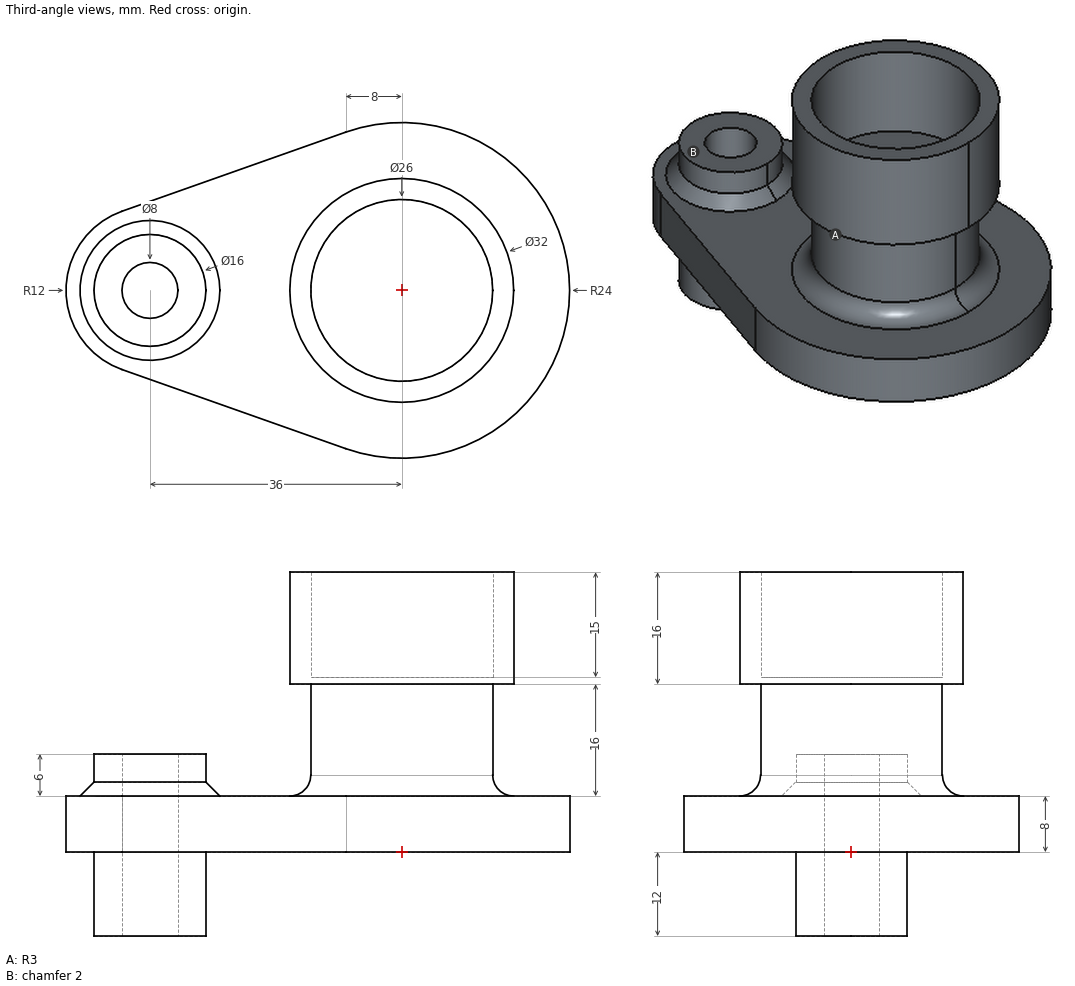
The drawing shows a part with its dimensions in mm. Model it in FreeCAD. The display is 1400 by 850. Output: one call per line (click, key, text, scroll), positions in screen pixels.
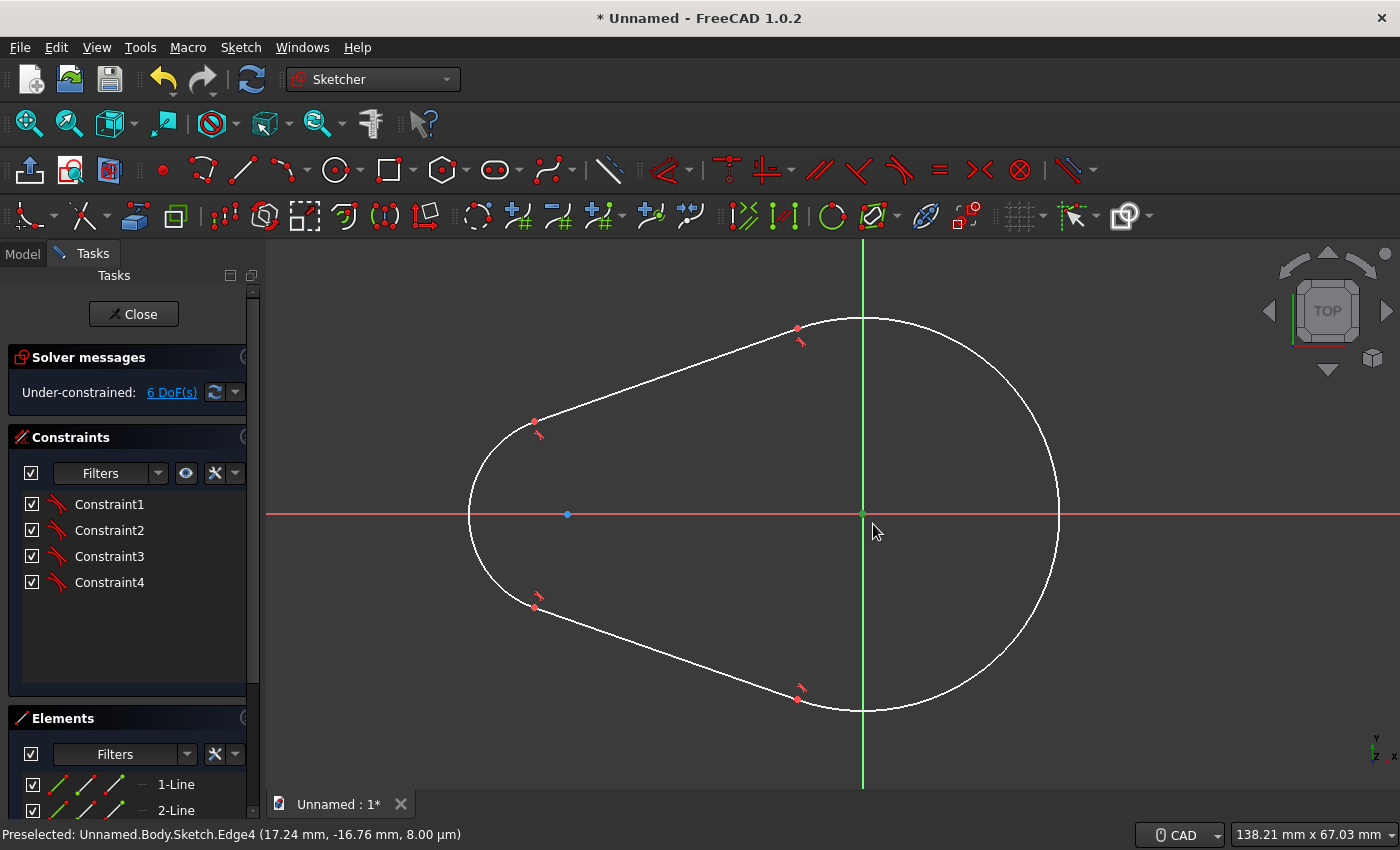
key(c)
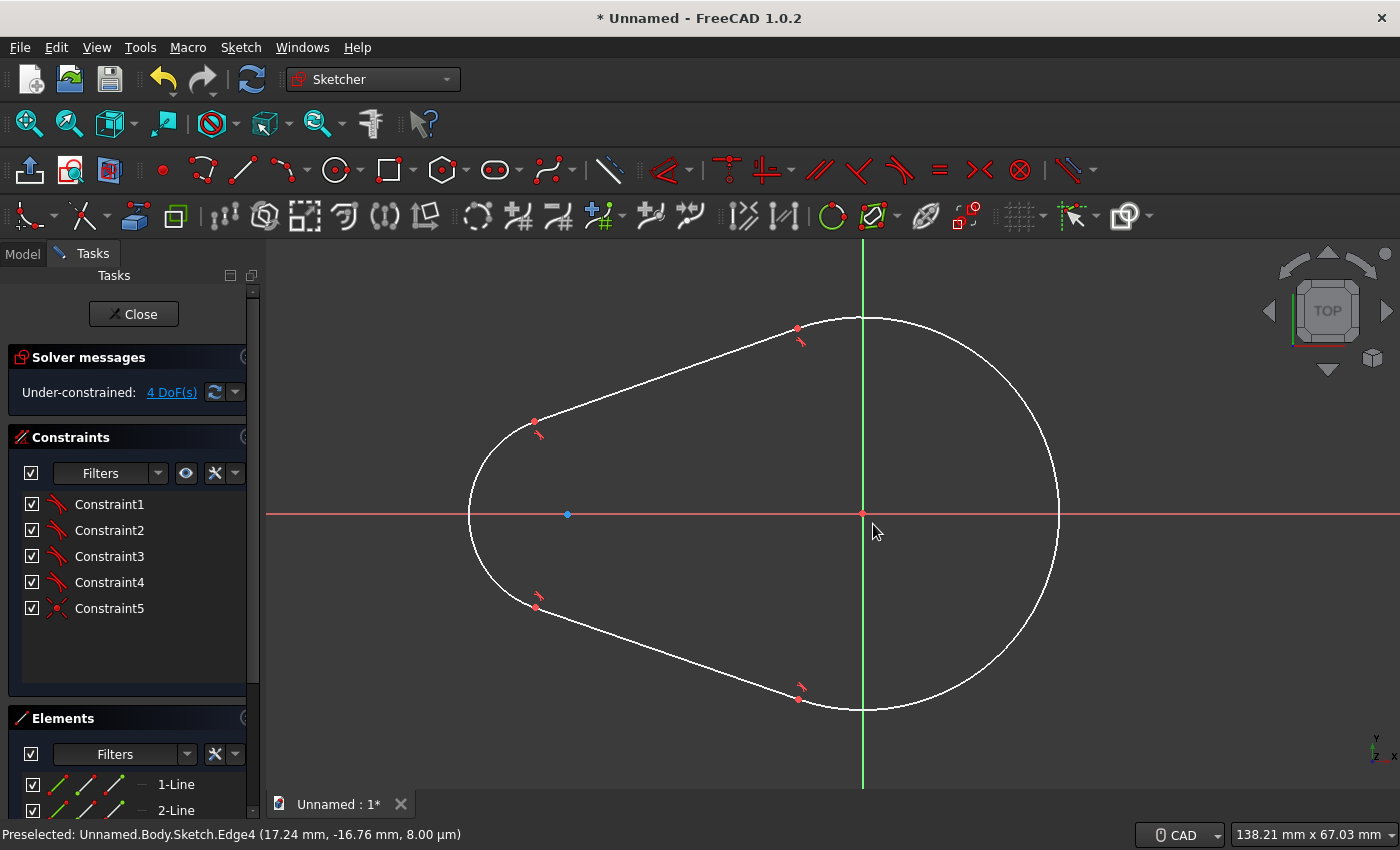
click(568, 515)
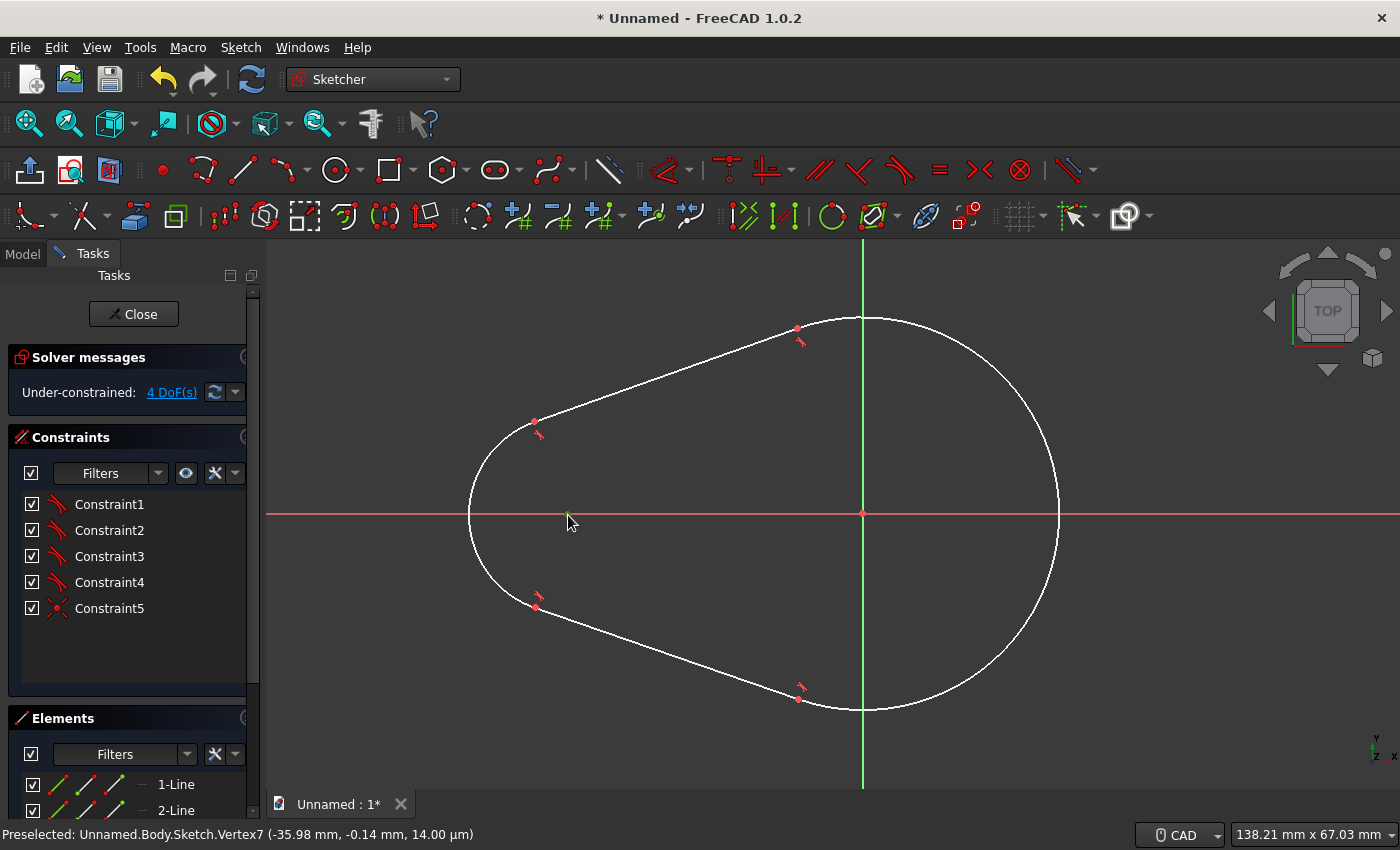
click(361, 514)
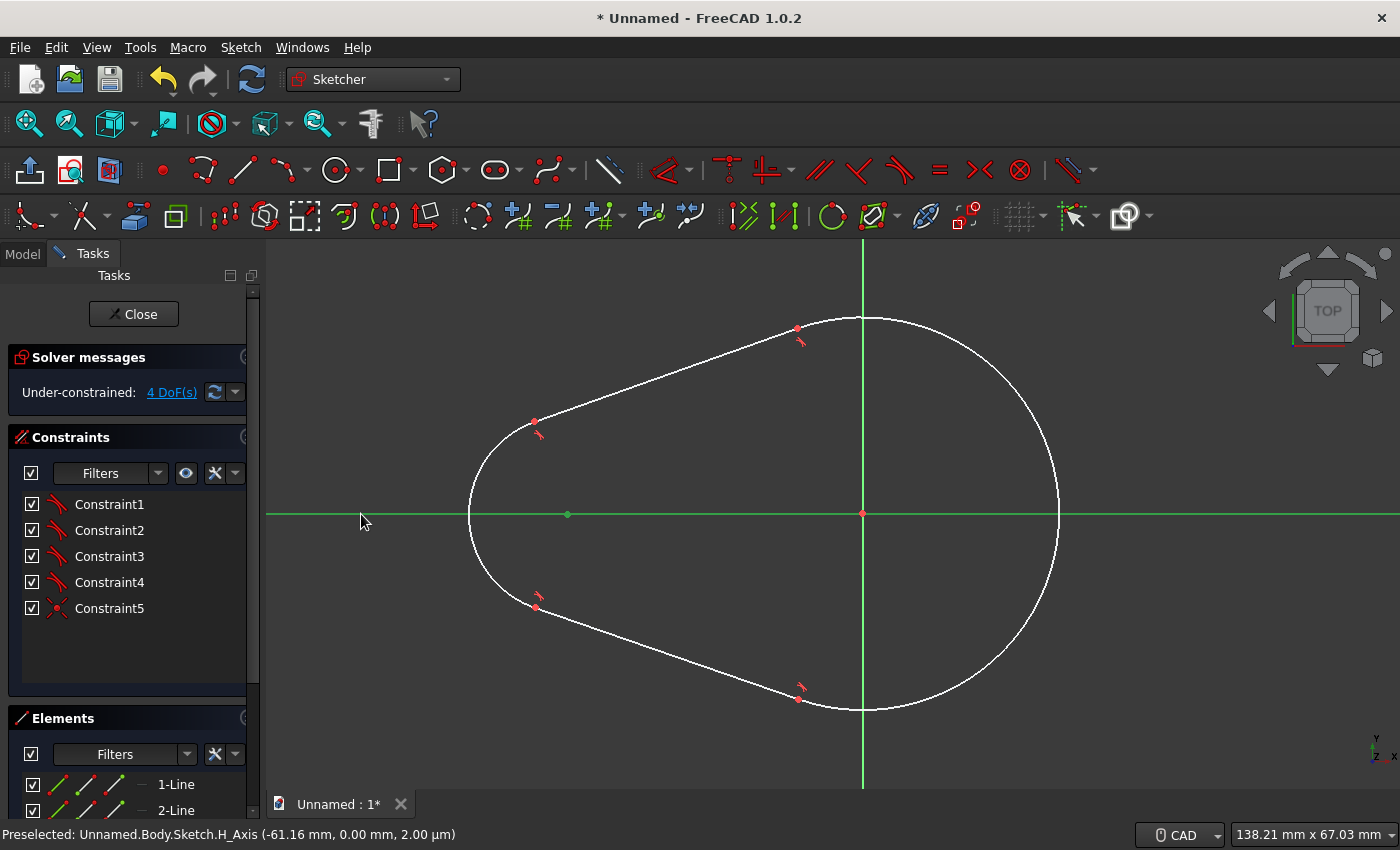
click(728, 170)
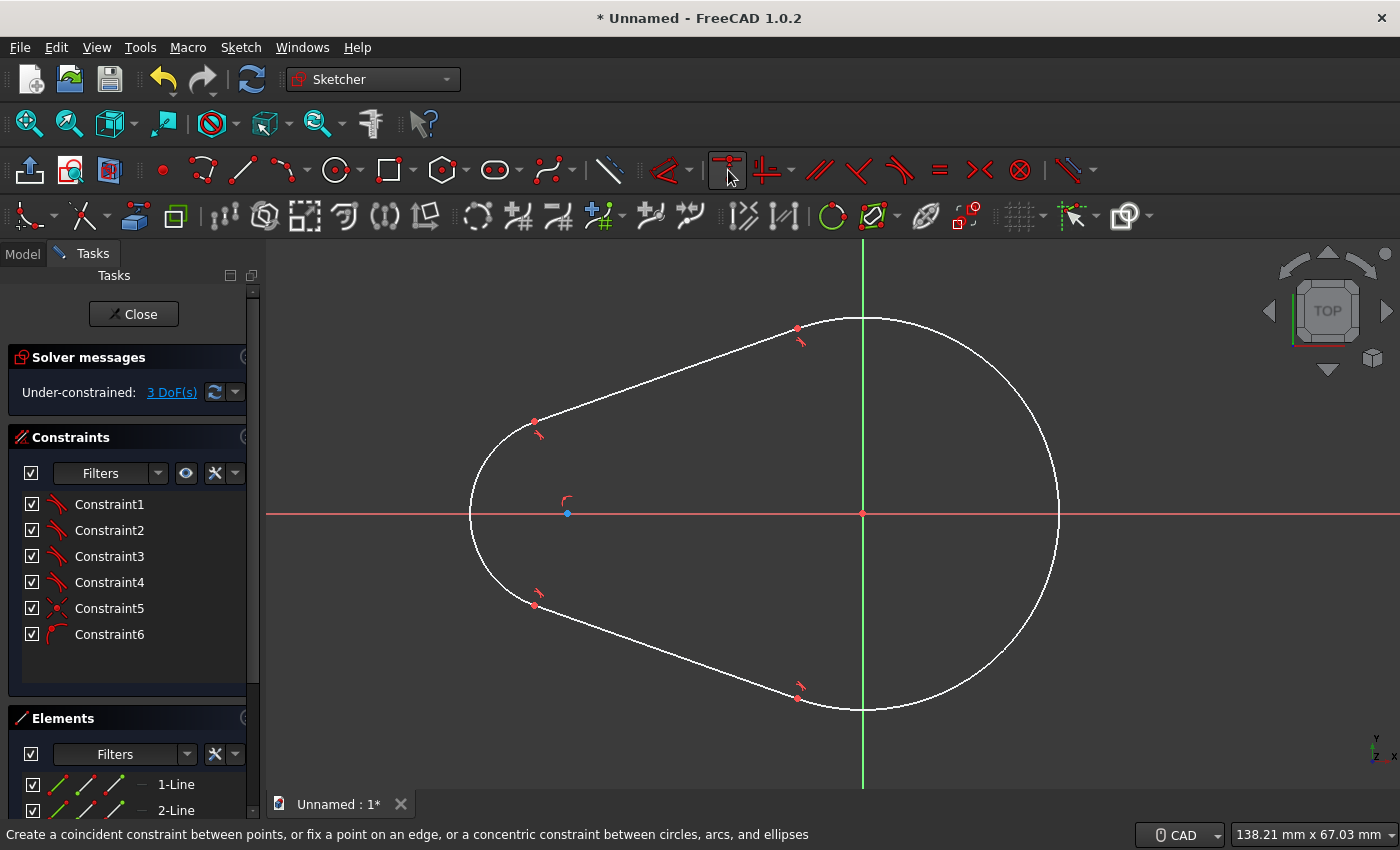
click(664, 170)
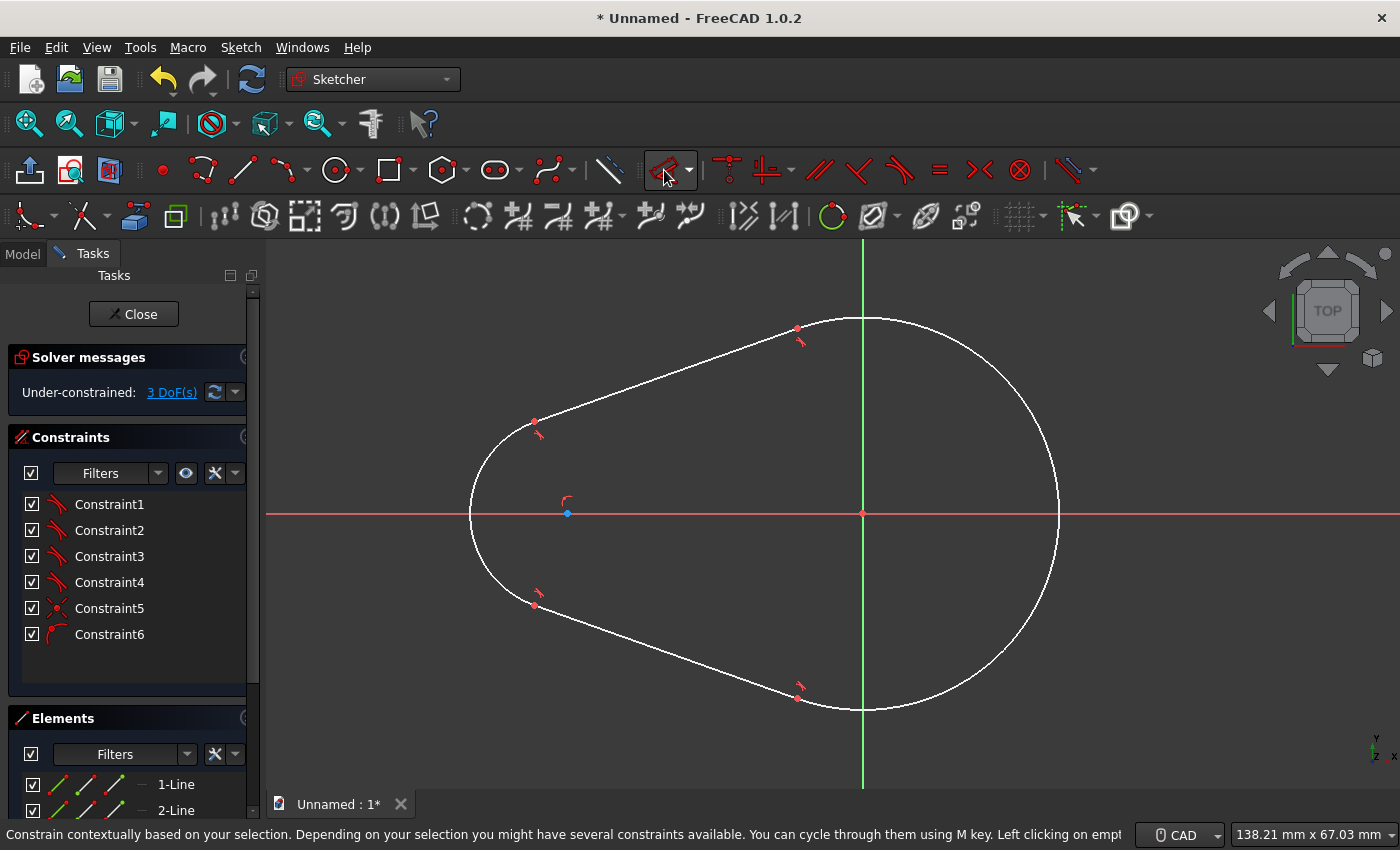
click(482, 468)
click(454, 453)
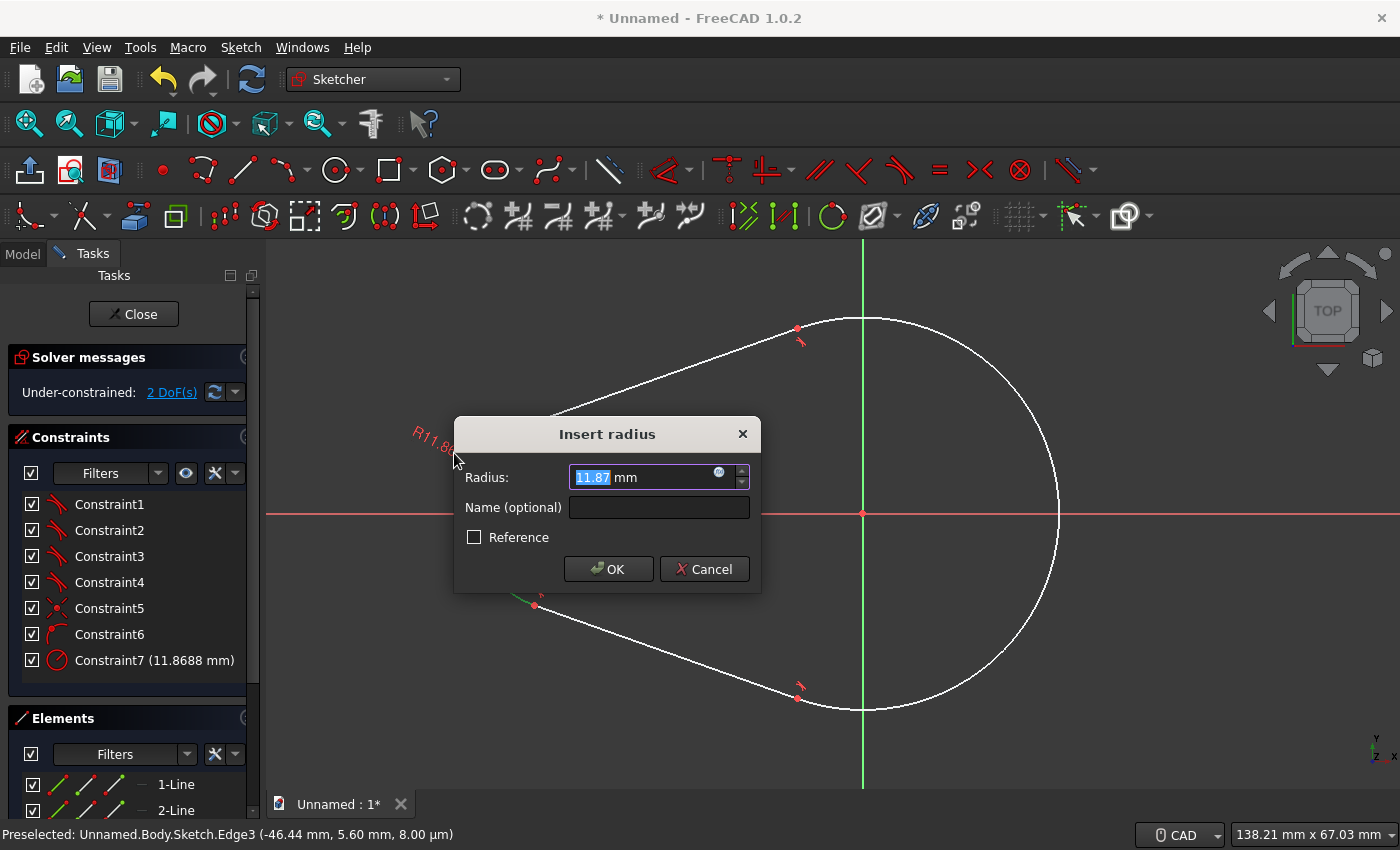
text(12)
key(Return)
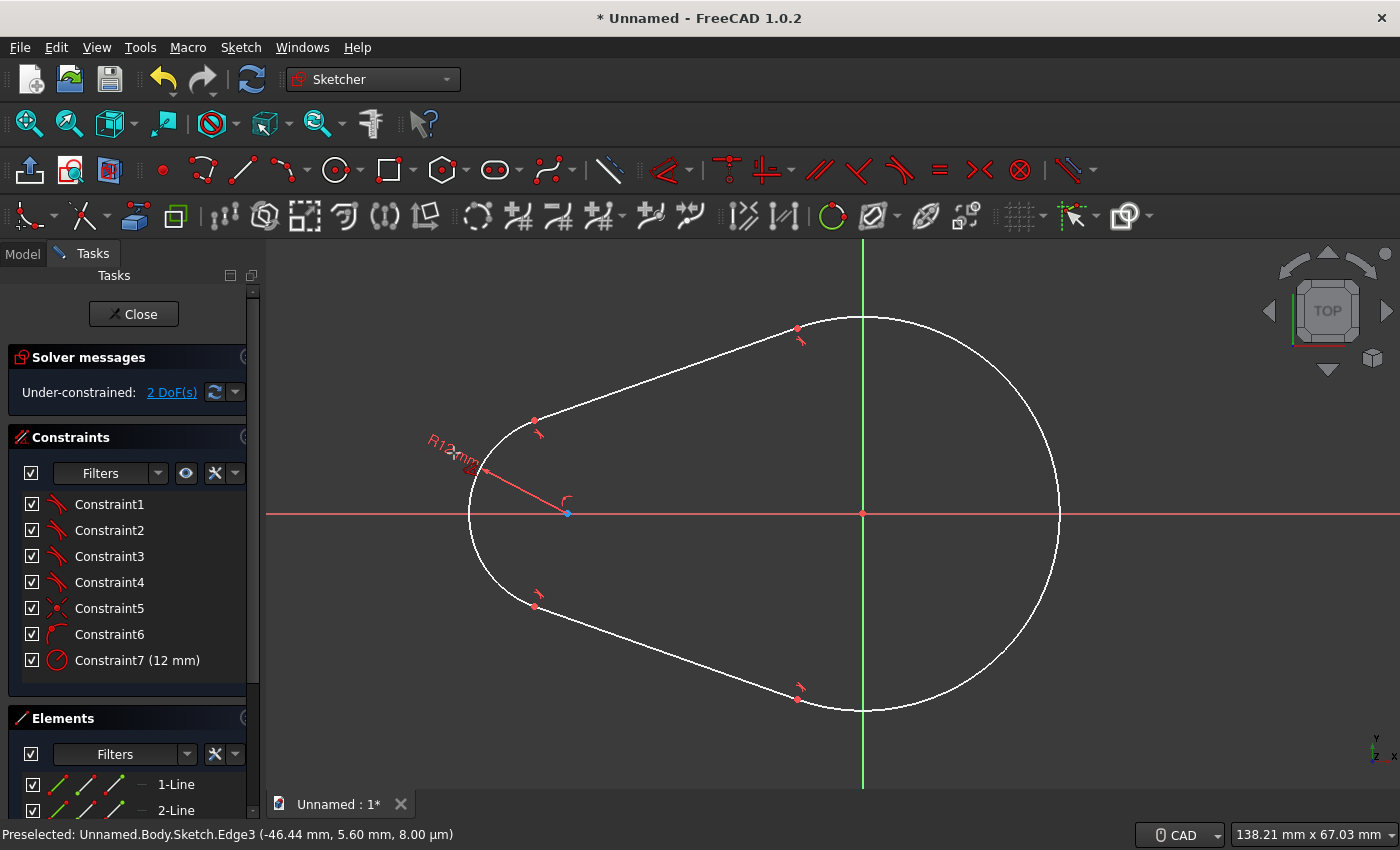
click(1005, 650)
click(1028, 672)